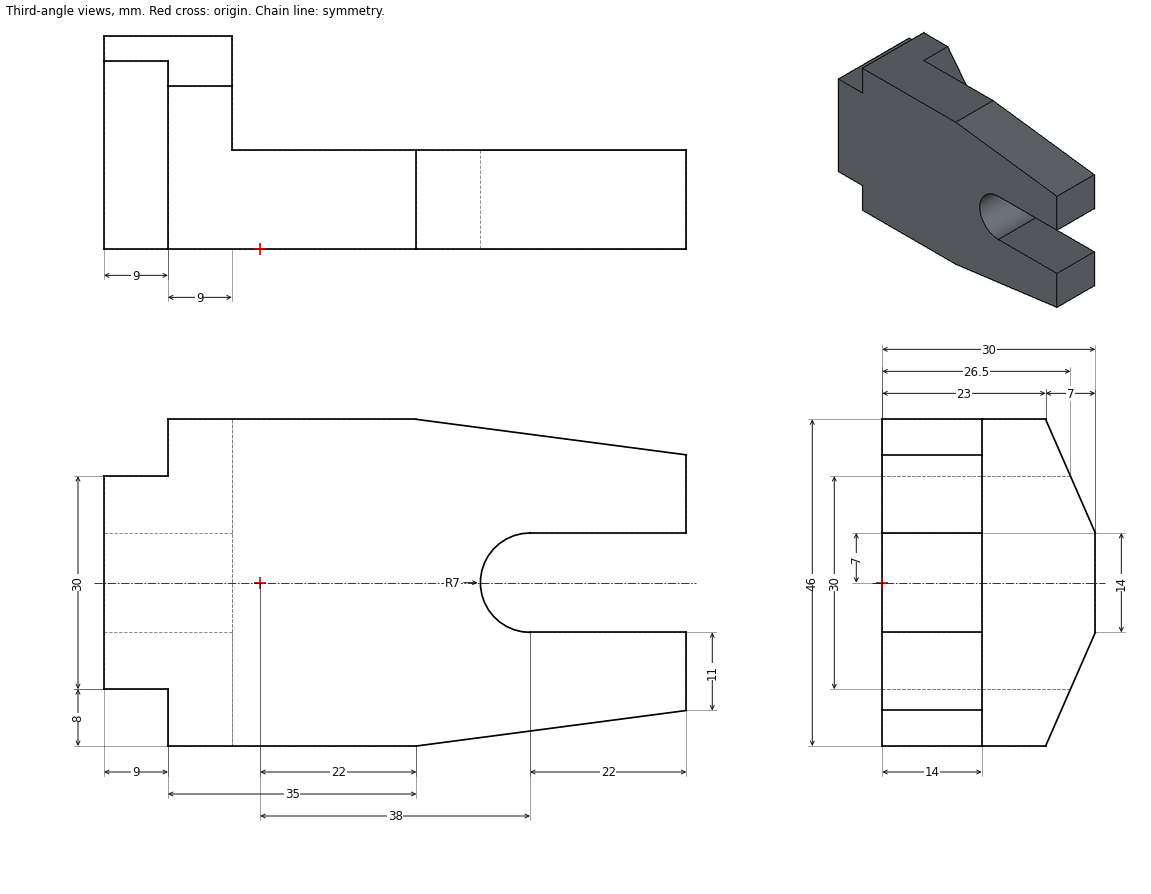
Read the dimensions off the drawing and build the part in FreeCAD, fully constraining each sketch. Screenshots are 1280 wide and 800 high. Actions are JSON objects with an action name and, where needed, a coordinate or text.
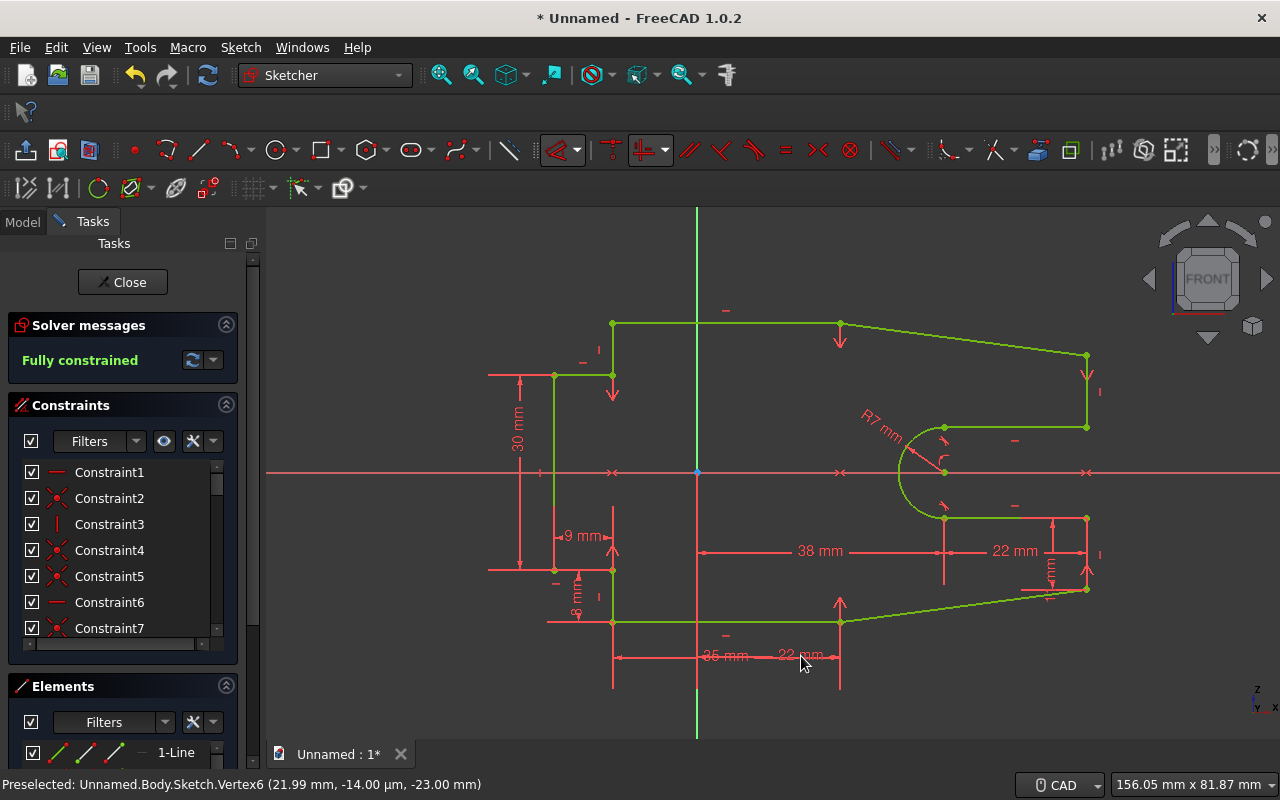
{"action": "left_click", "coordinate": [123, 282]}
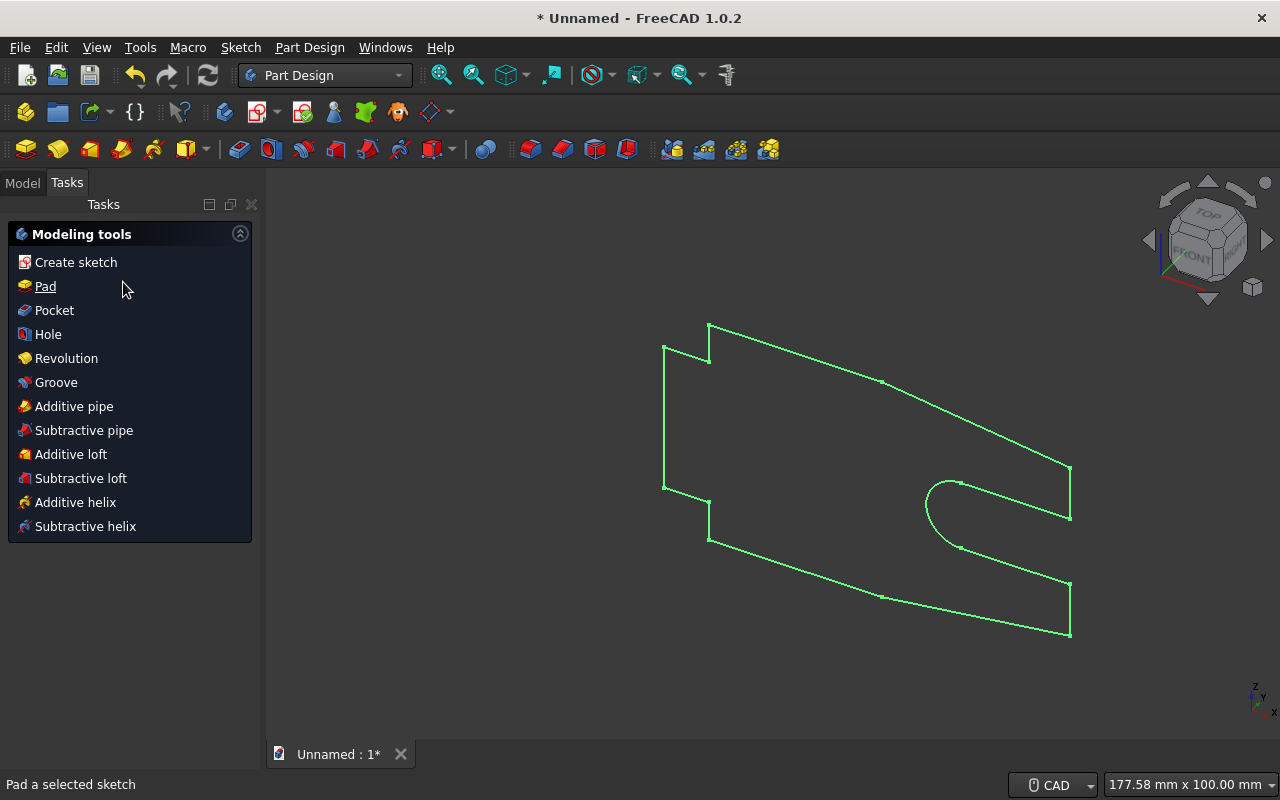
{"action": "left_click", "coordinate": [26, 150]}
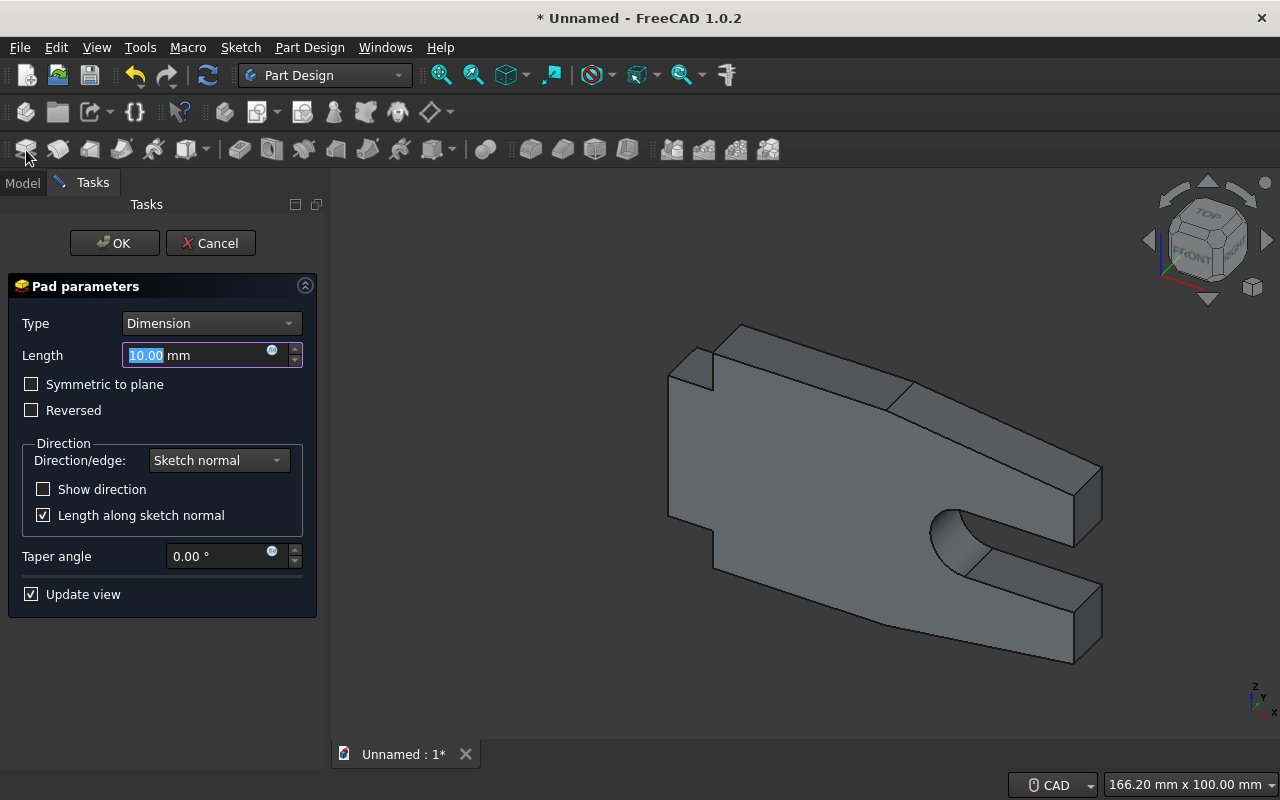
{"action": "type", "text": "14"}
{"action": "key", "text": "Tab"}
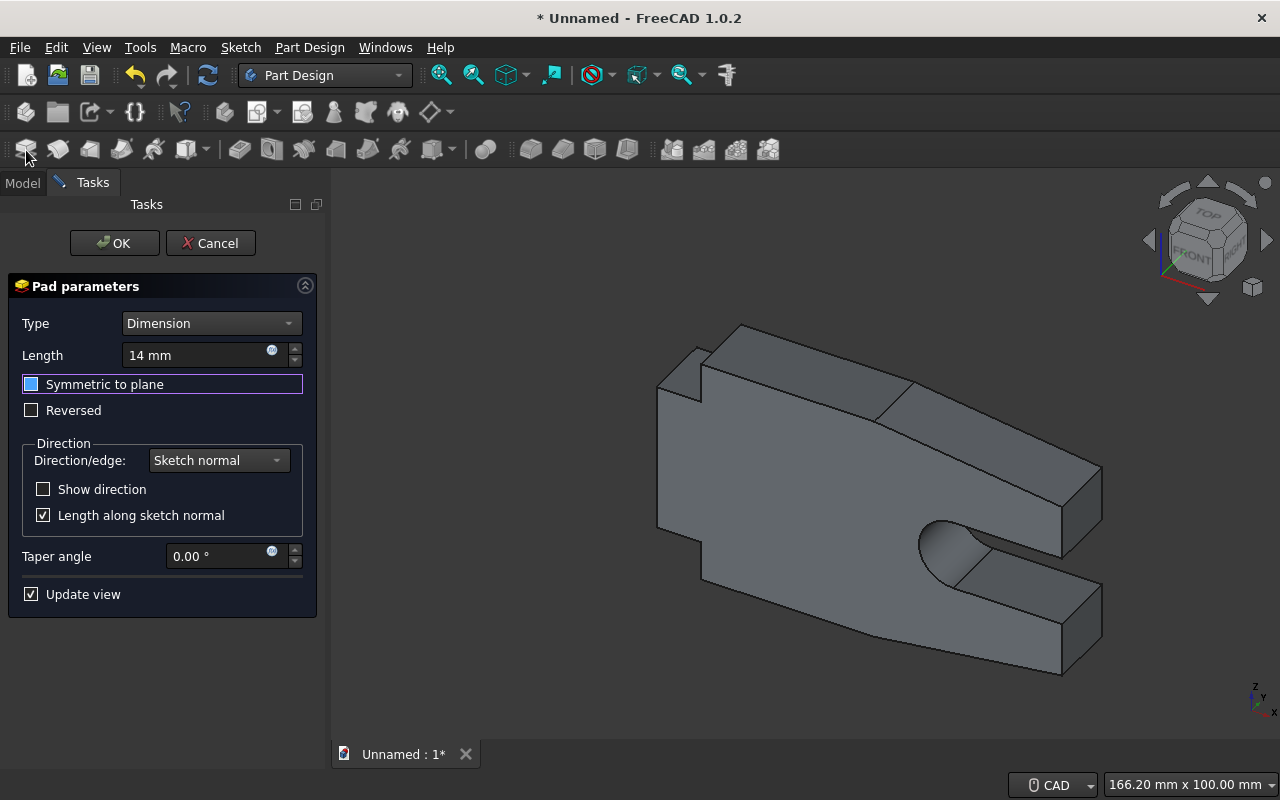
{"action": "left_click", "coordinate": [30, 410]}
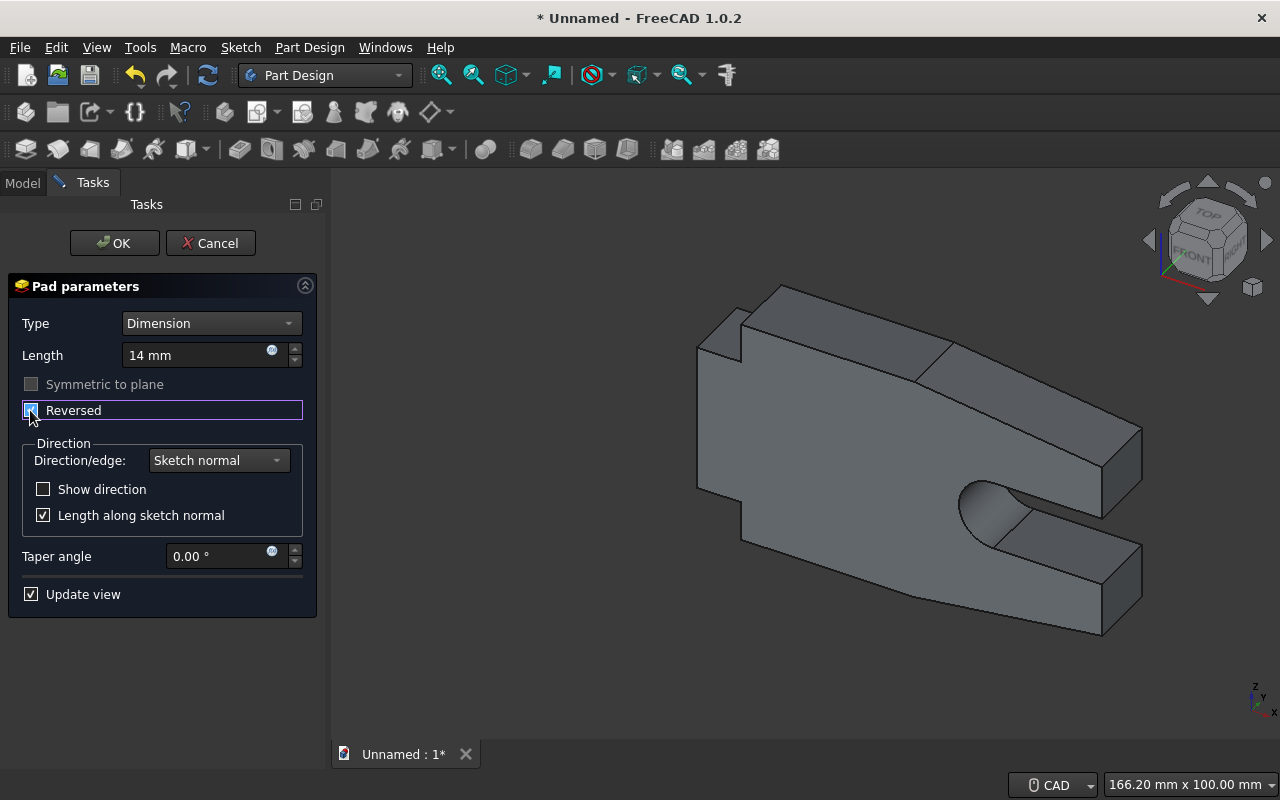
{"action": "left_click", "coordinate": [115, 243]}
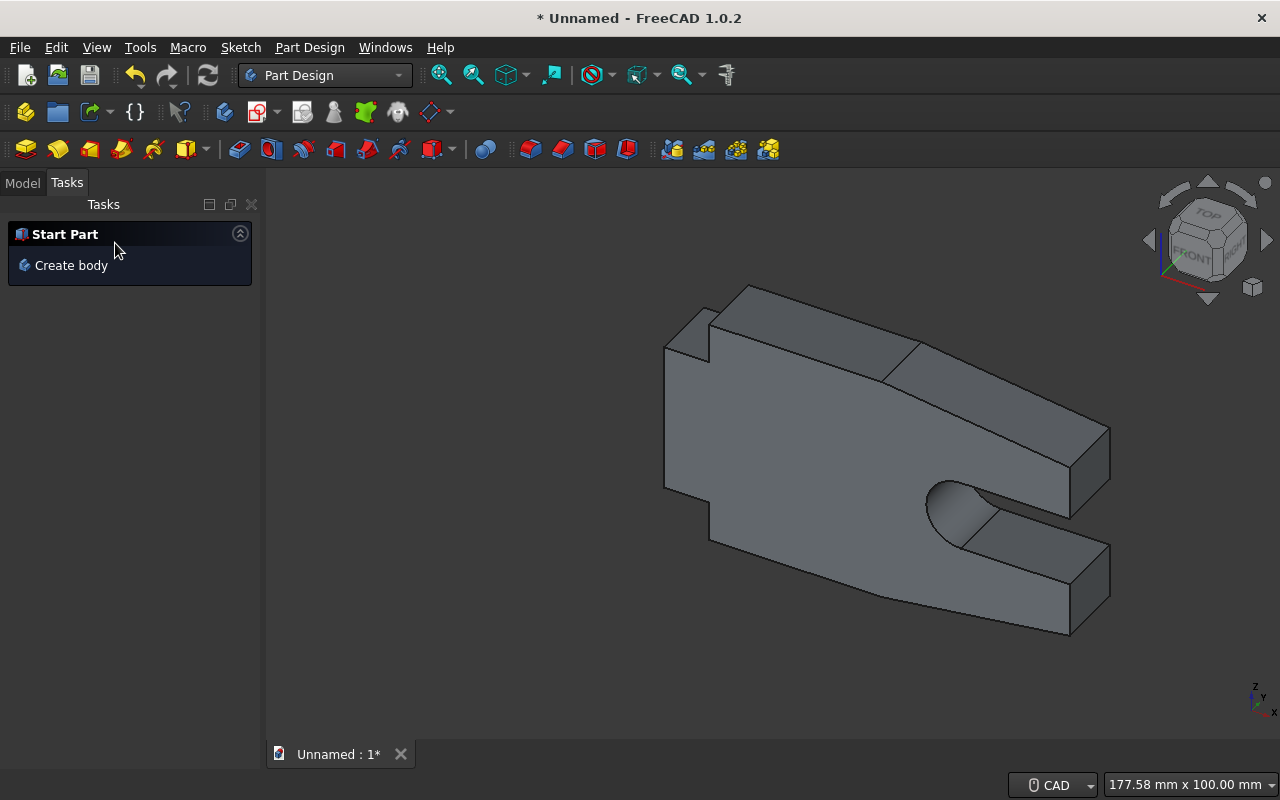
{"action": "key", "text": "6"}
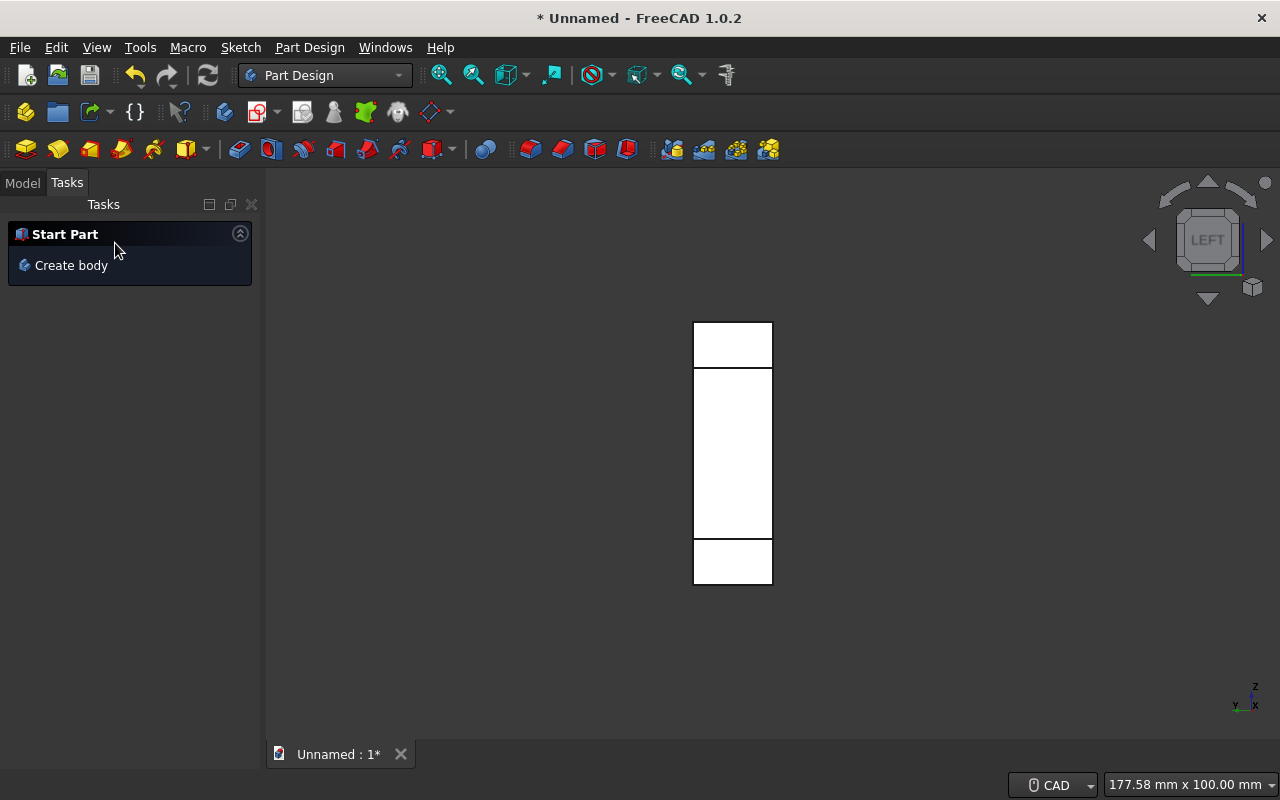
{"action": "left_click", "coordinate": [733, 452]}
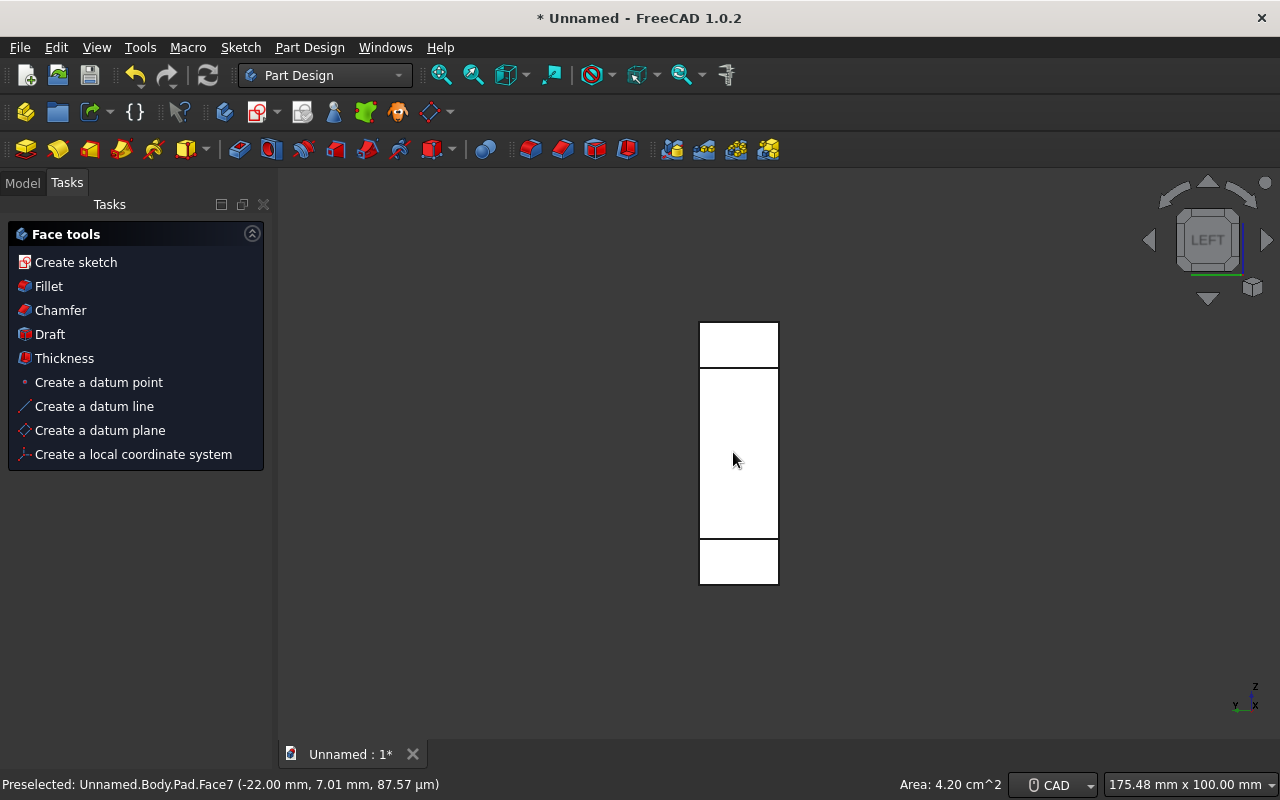
{"action": "left_click", "coordinate": [258, 112]}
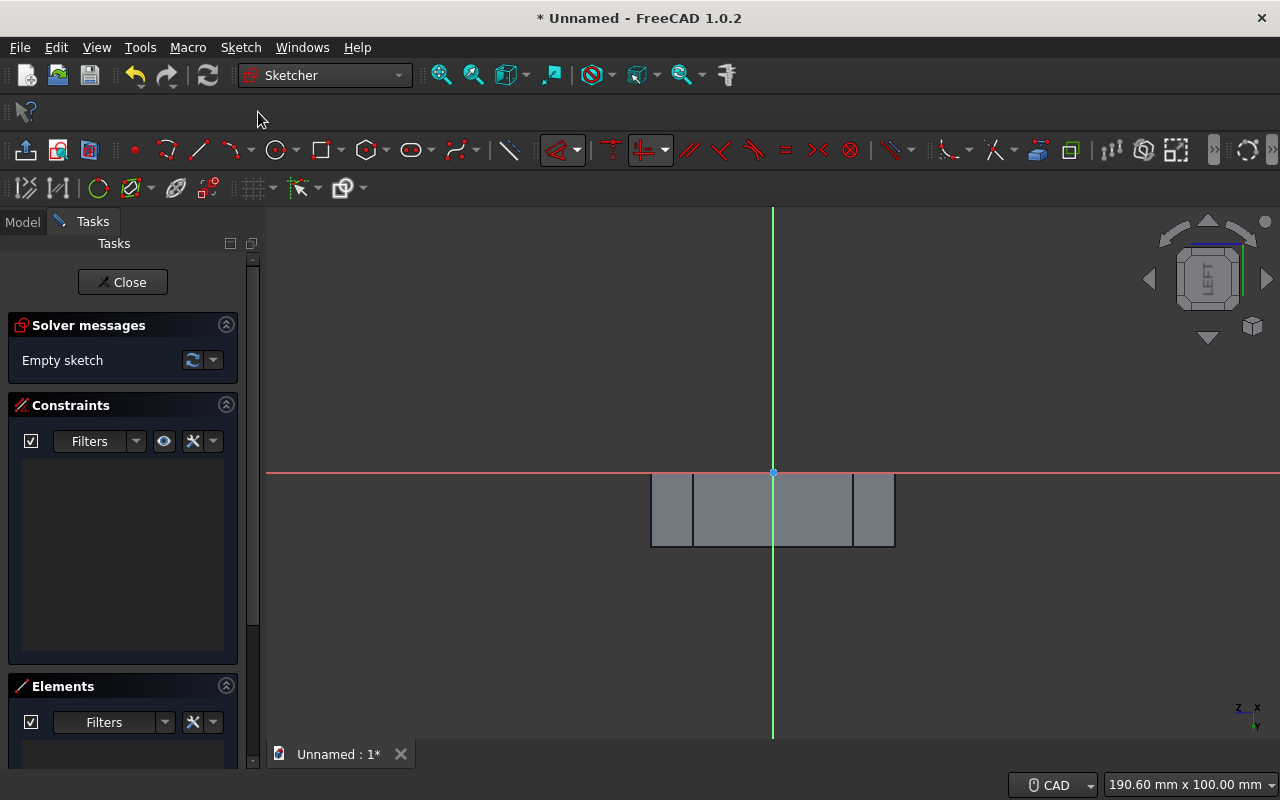
{"action": "scroll", "coordinate": [829, 618], "scroll_direction": "up", "scroll_amount": 4}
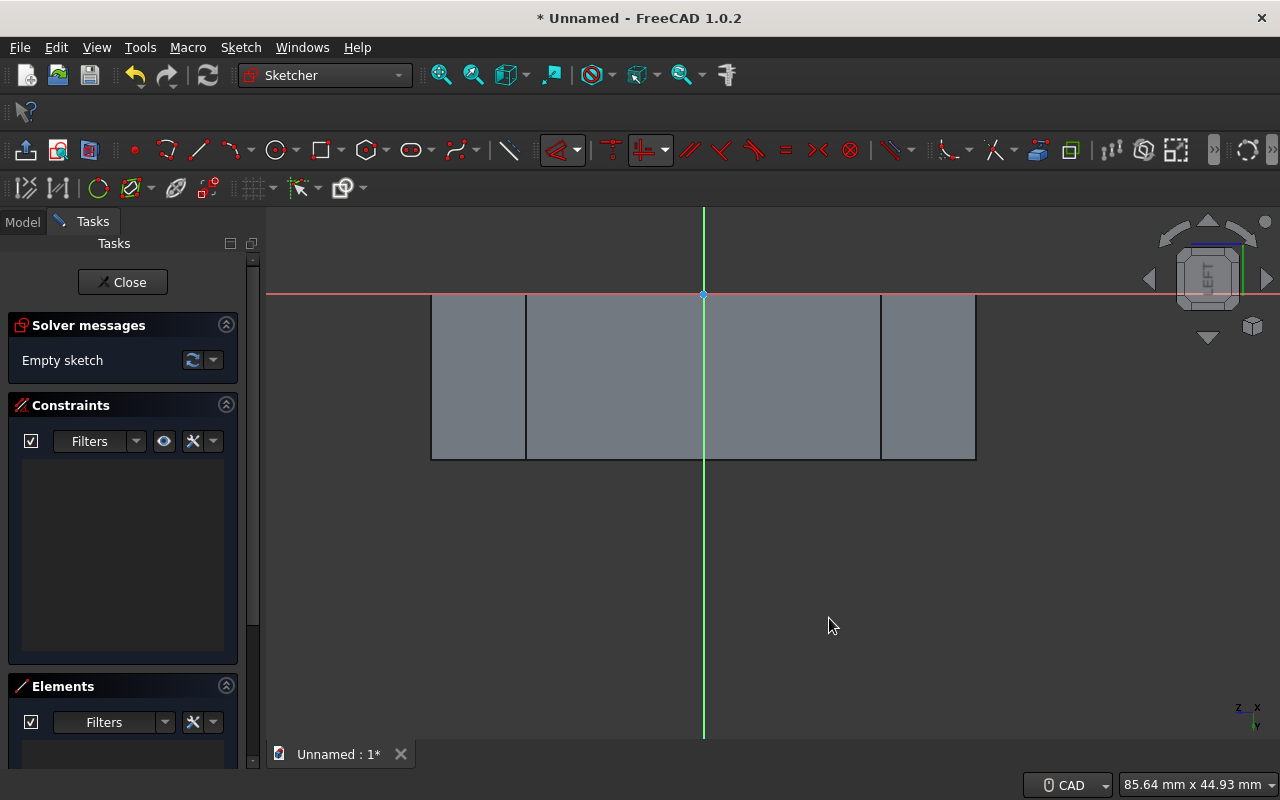
{"action": "key", "text": "g m"}